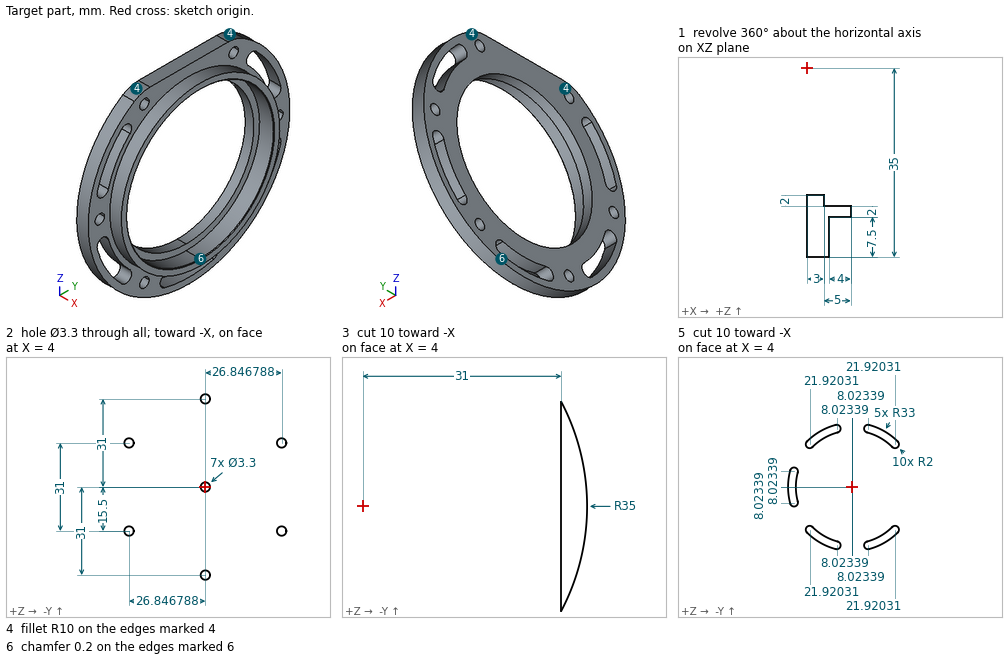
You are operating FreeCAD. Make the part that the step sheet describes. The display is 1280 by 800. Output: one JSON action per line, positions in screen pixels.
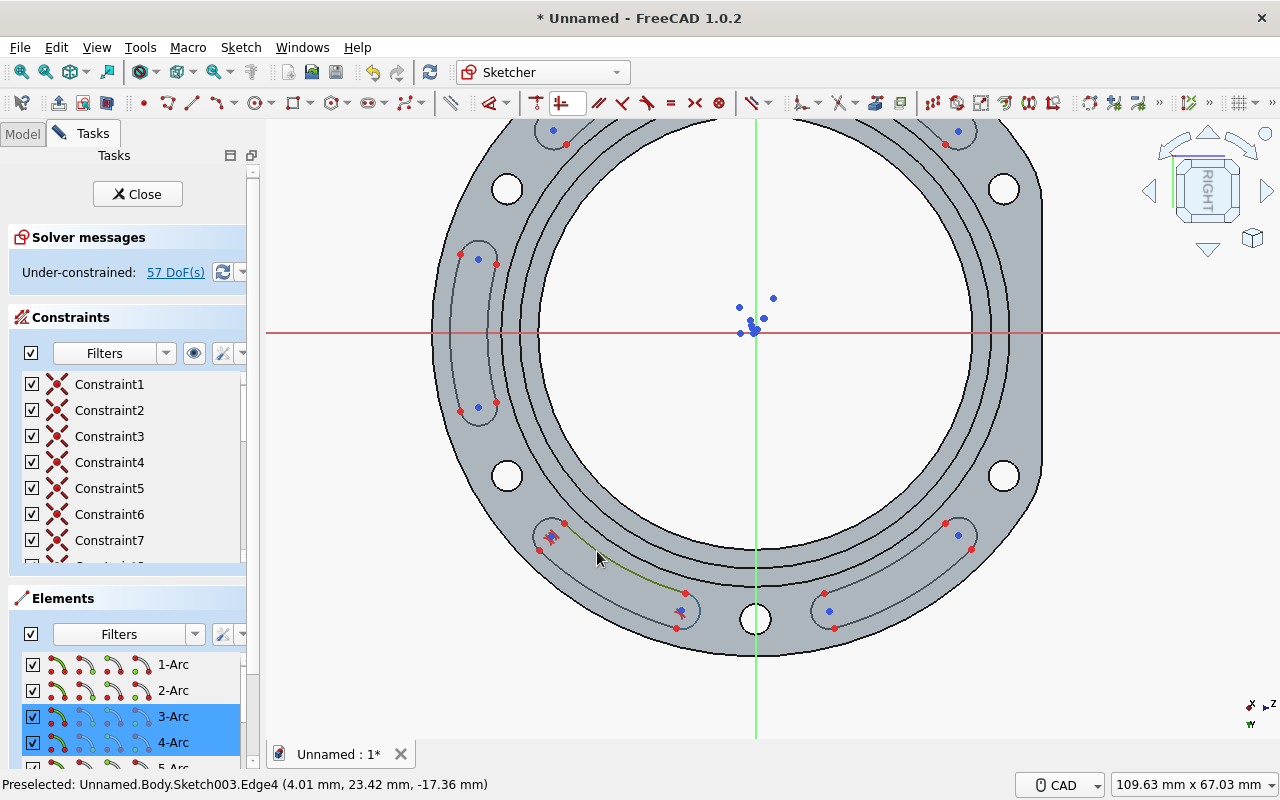
{"action": "left_click", "coordinate": [648, 104]}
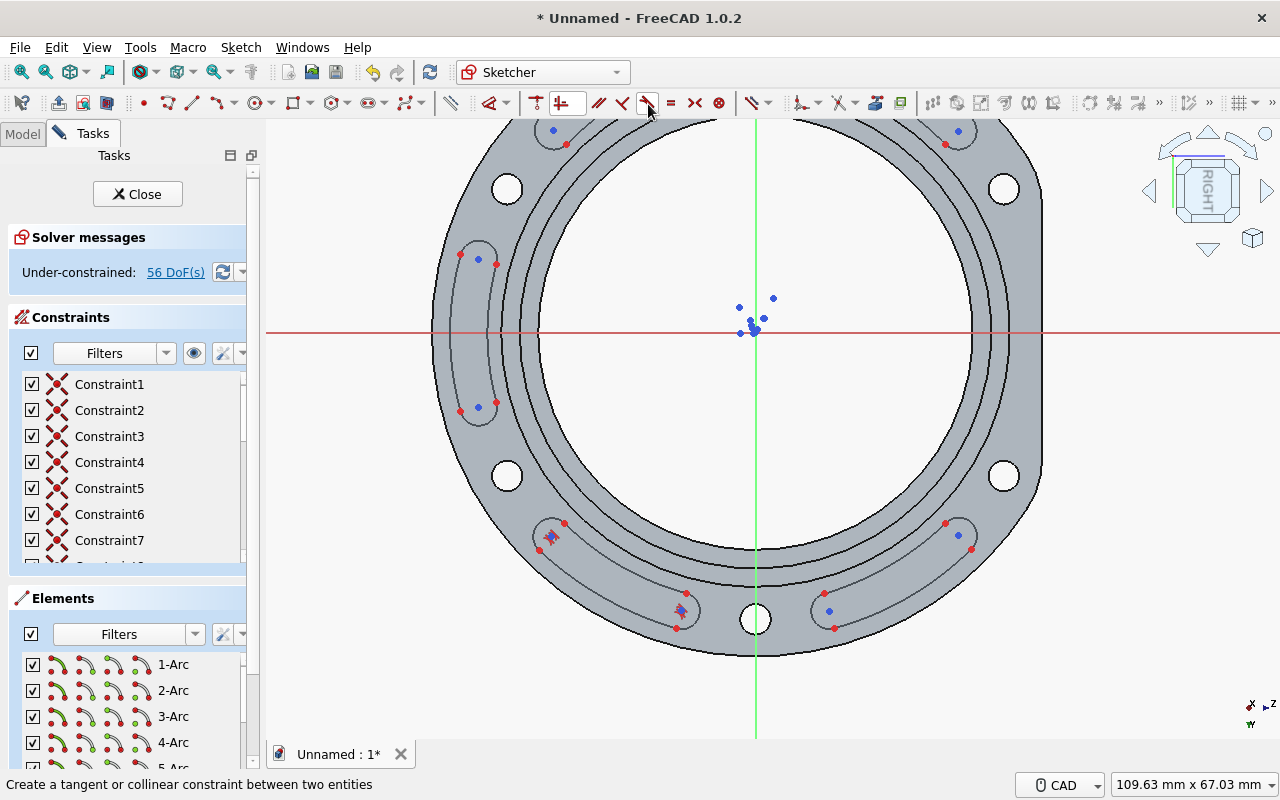
{"action": "left_click", "coordinate": [489, 306]}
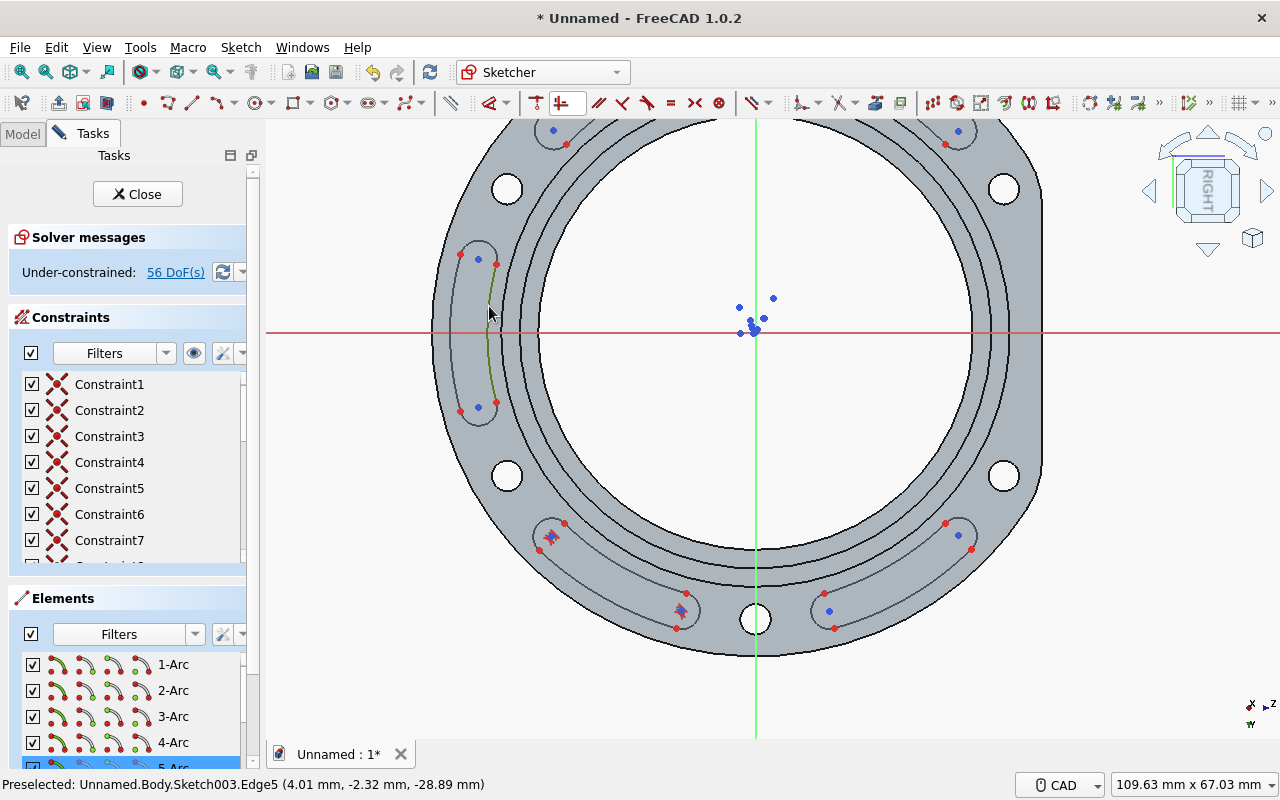
{"action": "left_click", "coordinate": [493, 248]}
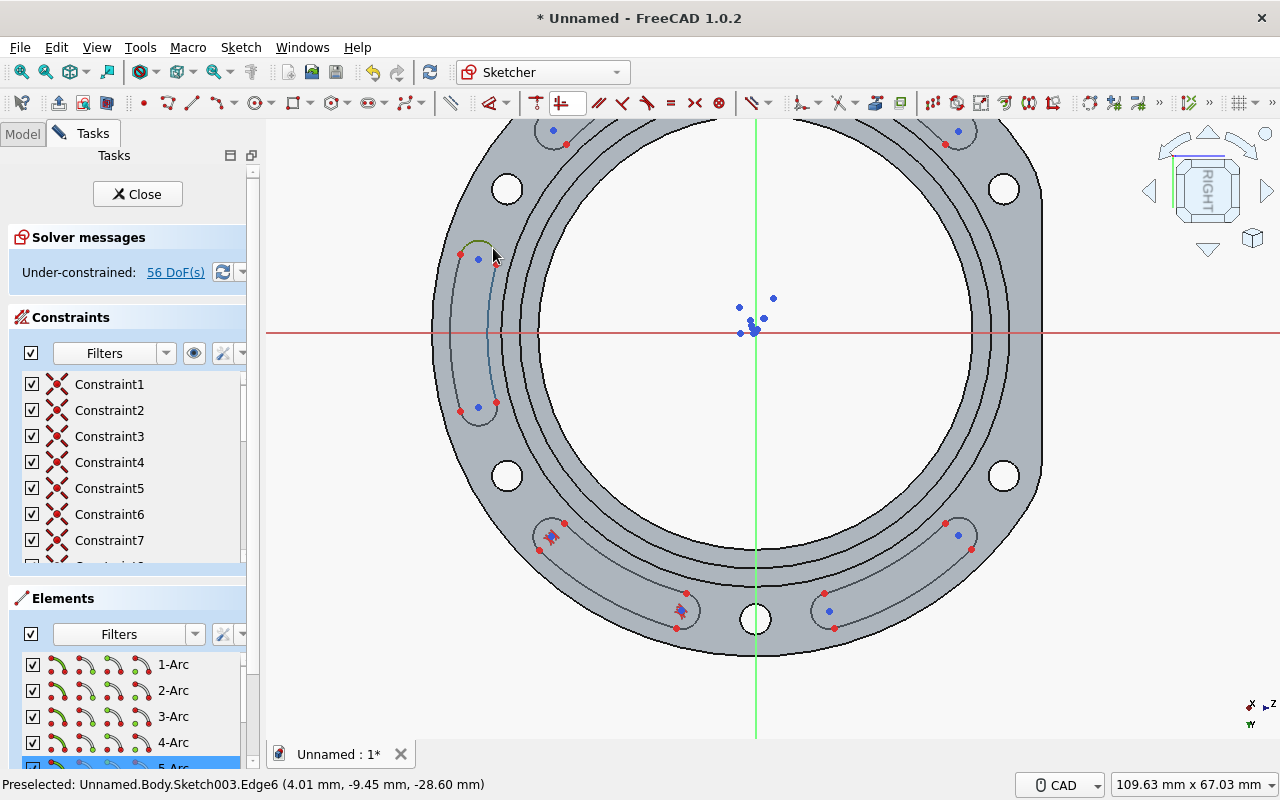
{"action": "left_click", "coordinate": [648, 104]}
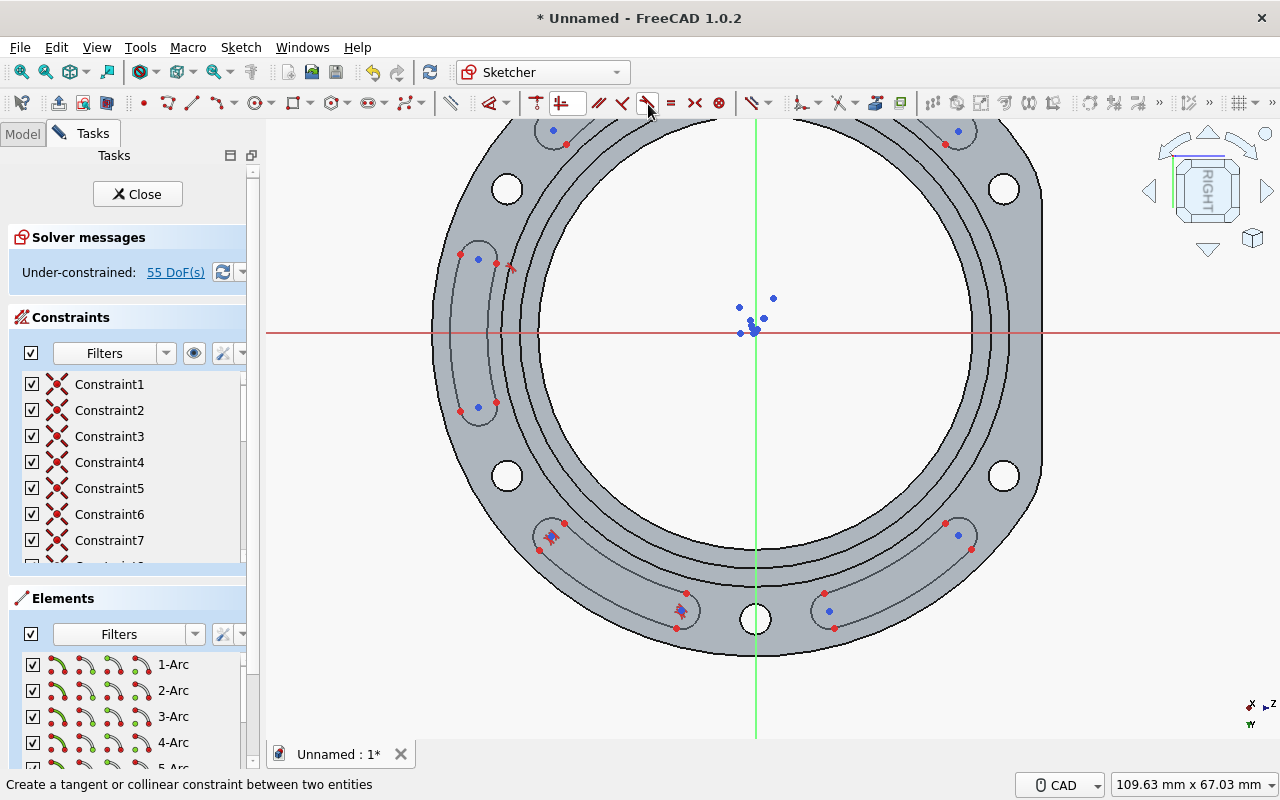
{"action": "left_click", "coordinate": [489, 305]}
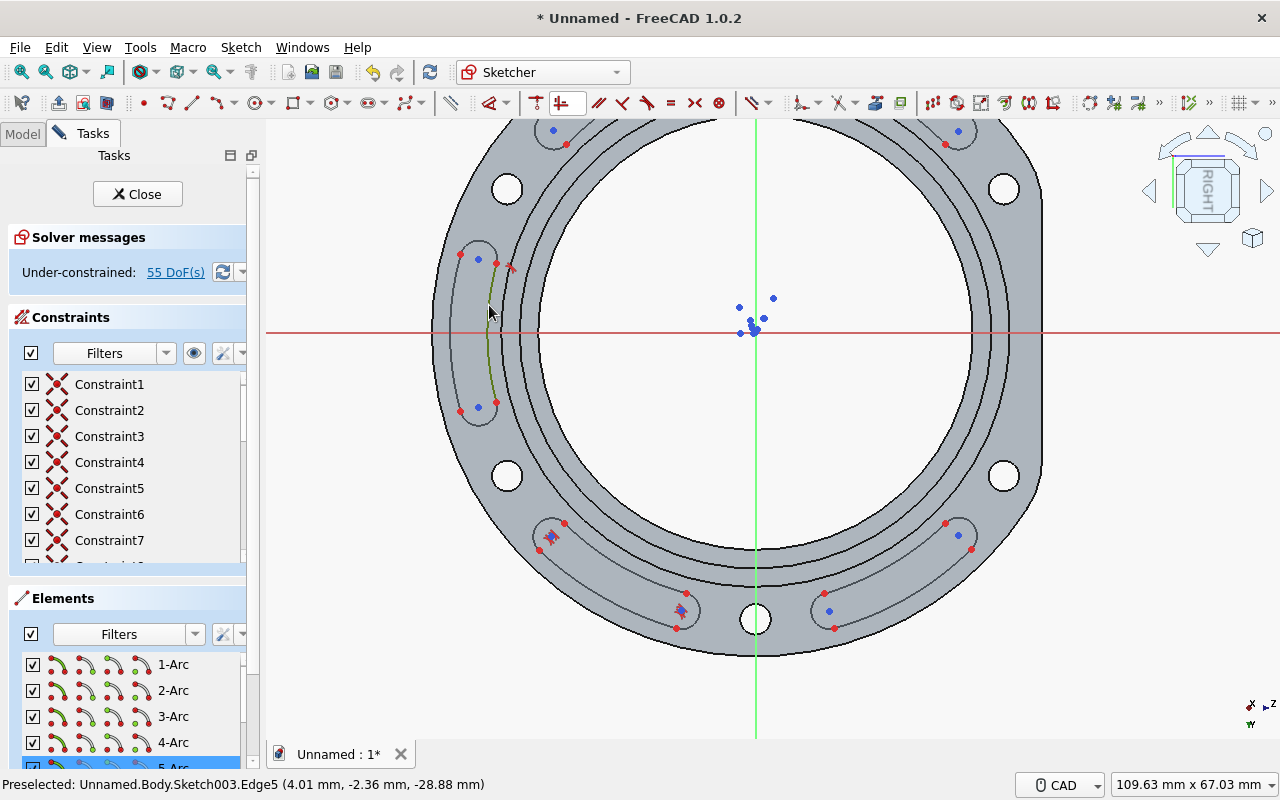
{"action": "left_click", "coordinate": [472, 424]}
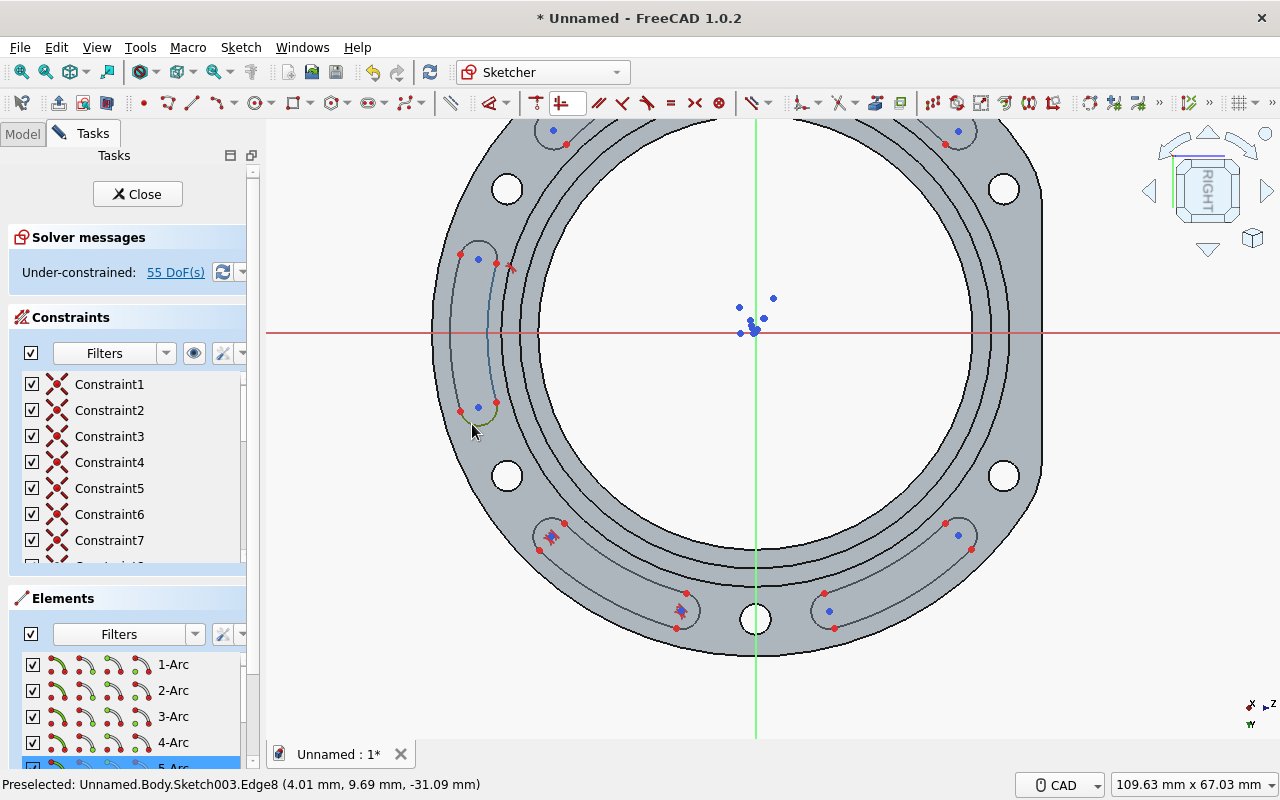
{"action": "left_click", "coordinate": [648, 104]}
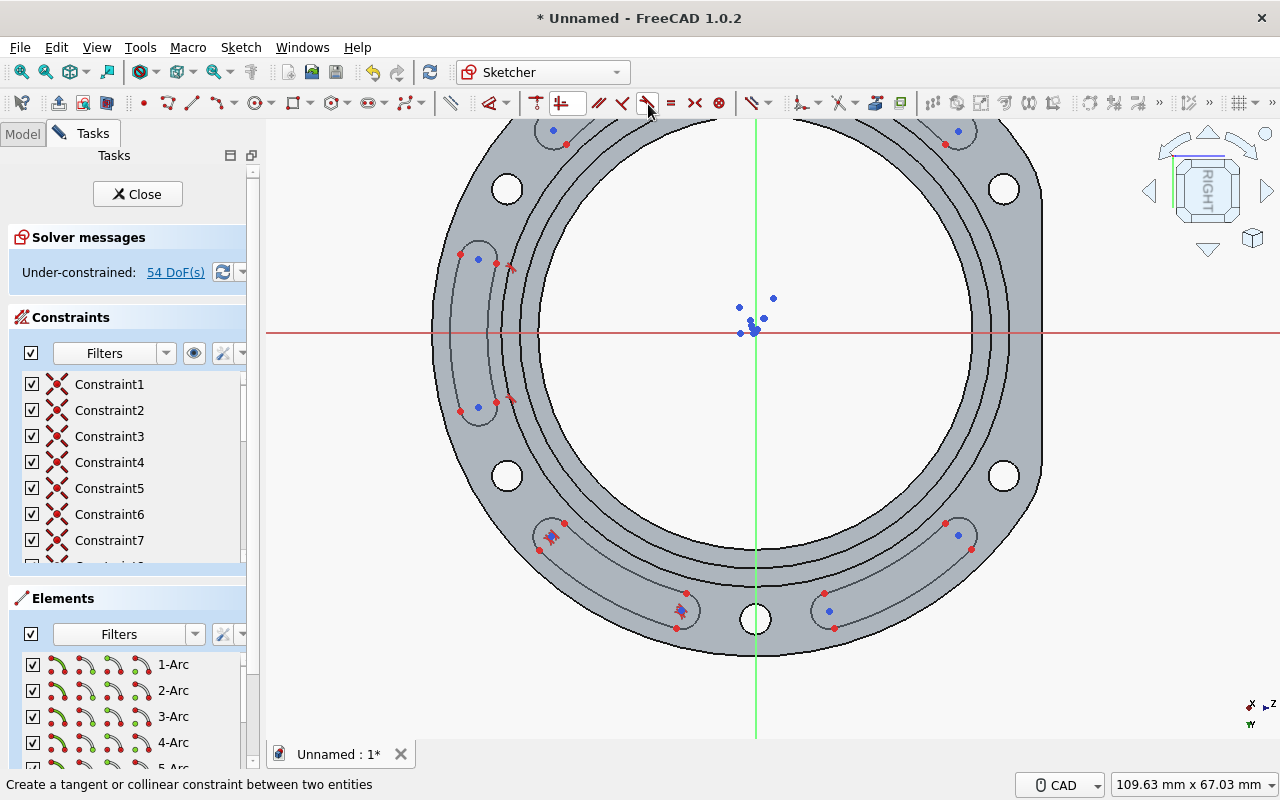
{"action": "left_click", "coordinate": [493, 248]}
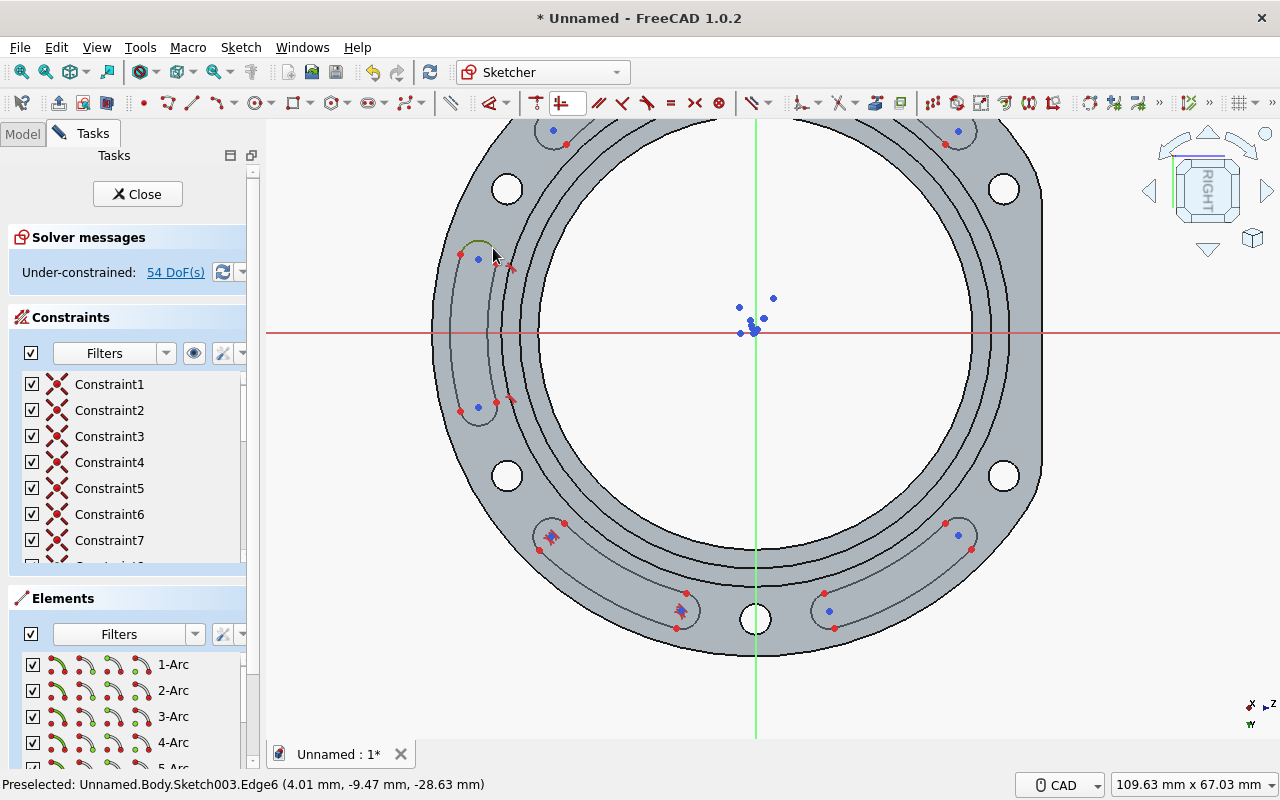
{"action": "left_click", "coordinate": [452, 301]}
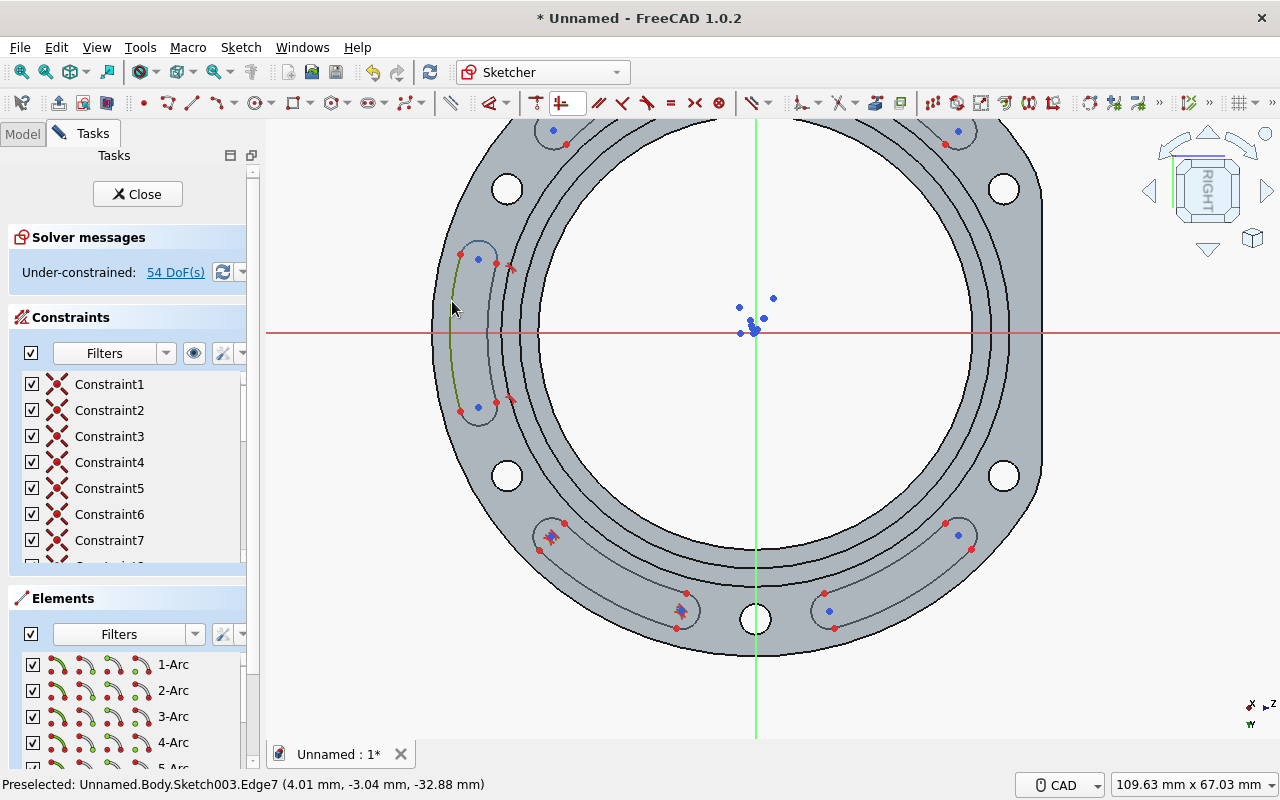
{"action": "left_click", "coordinate": [648, 104]}